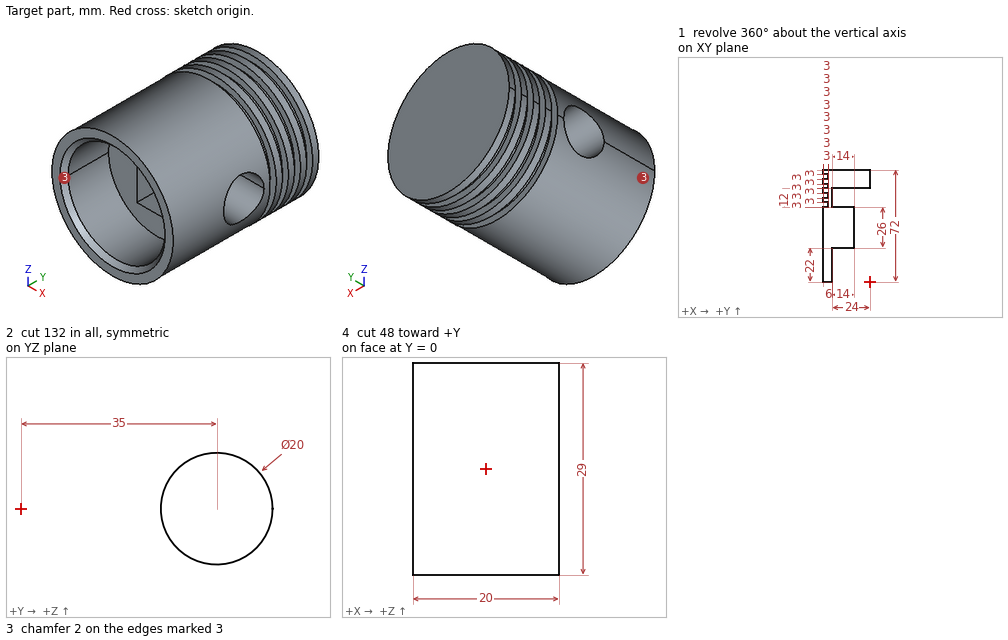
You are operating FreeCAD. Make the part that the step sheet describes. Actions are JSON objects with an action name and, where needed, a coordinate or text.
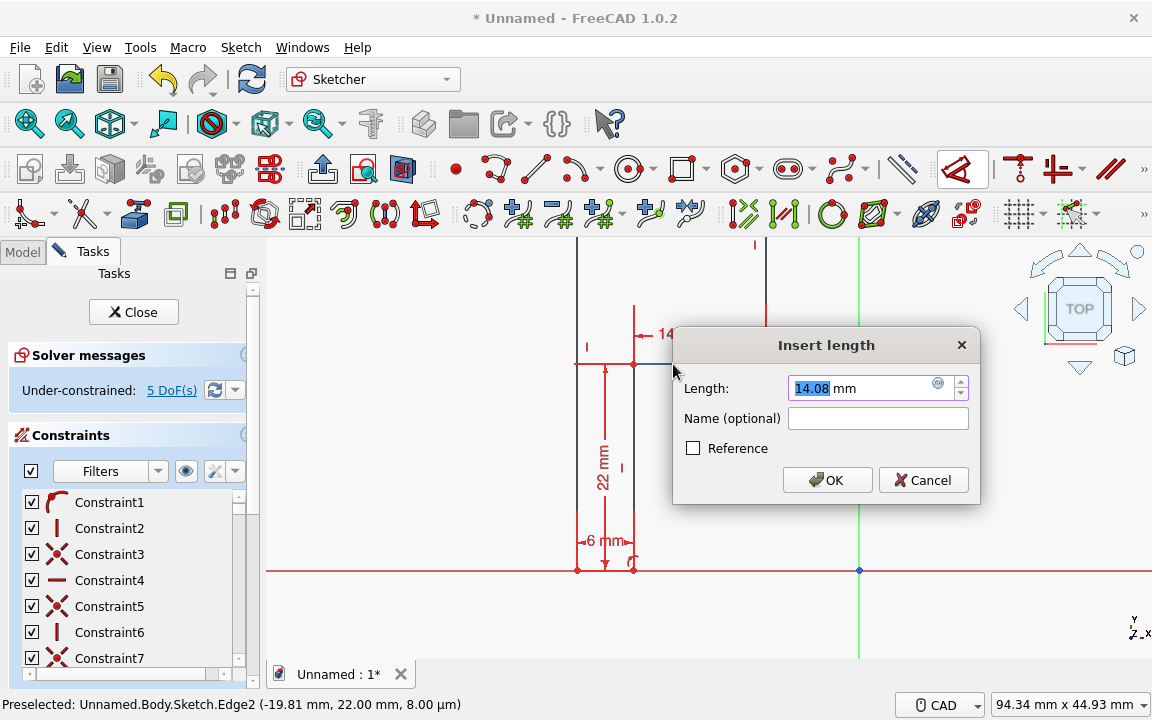
{"action": "type", "text": "14"}
{"action": "key", "text": "Return"}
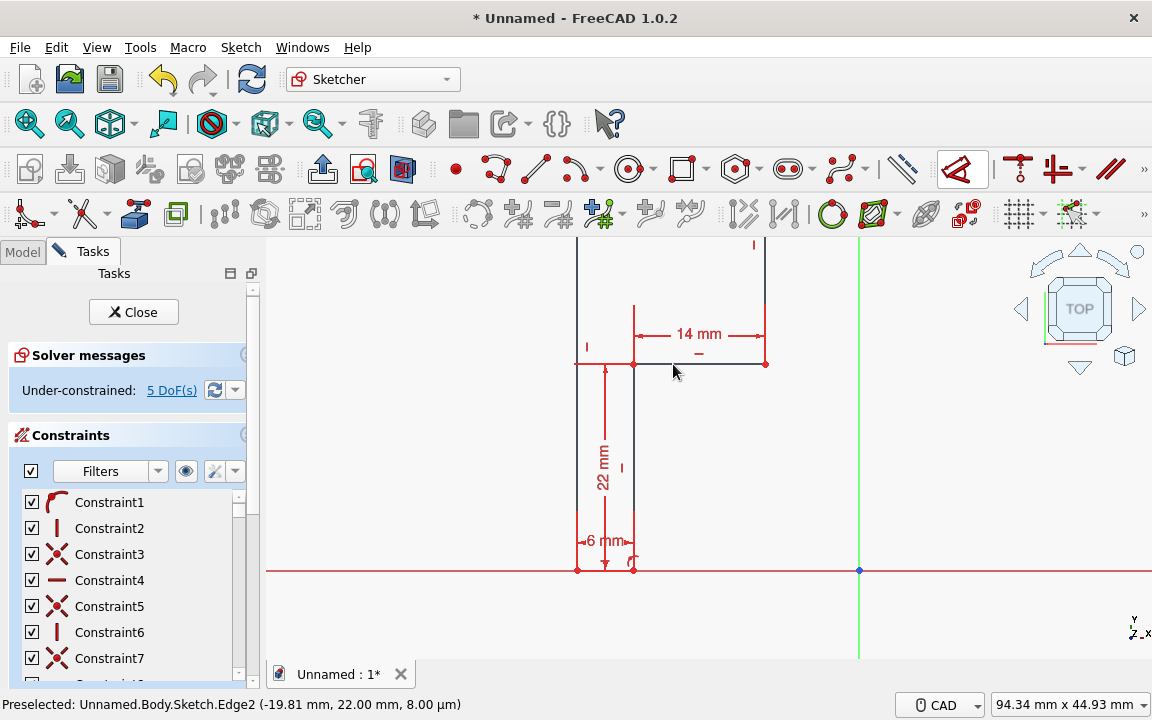
{"action": "left_click", "coordinate": [765, 292]}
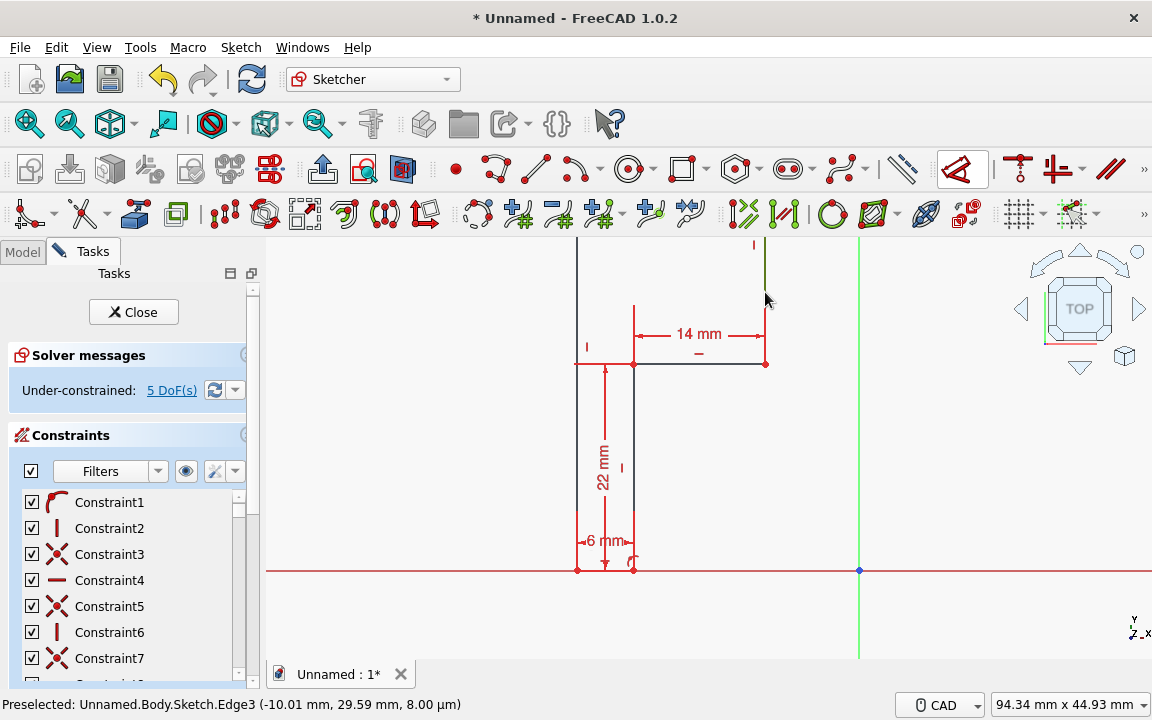
{"action": "left_click", "coordinate": [982, 170]}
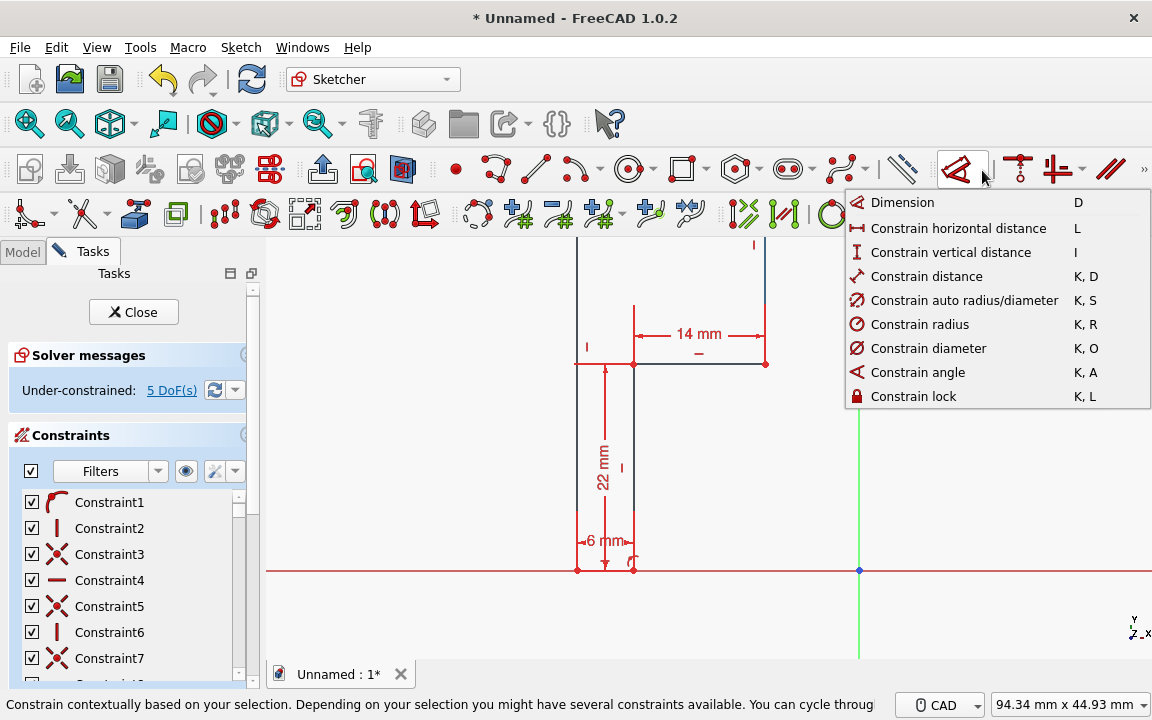
{"action": "left_click", "coordinate": [998, 252]}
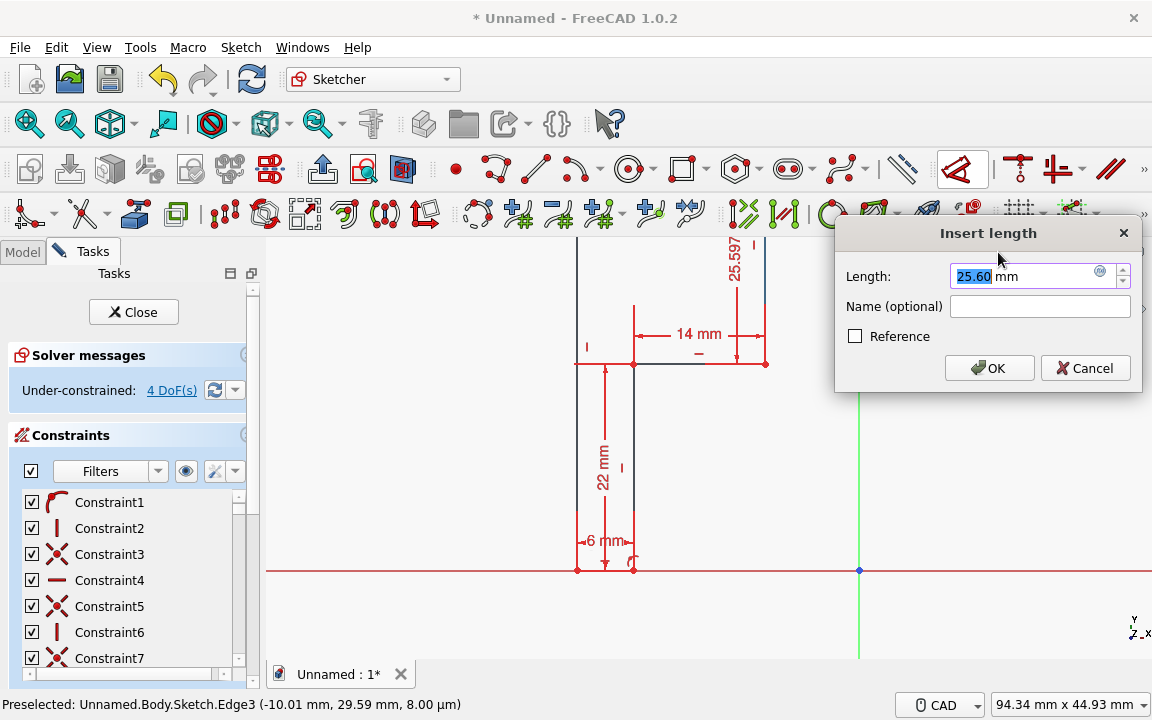
{"action": "type", "text": "26"}
{"action": "key", "text": "Return"}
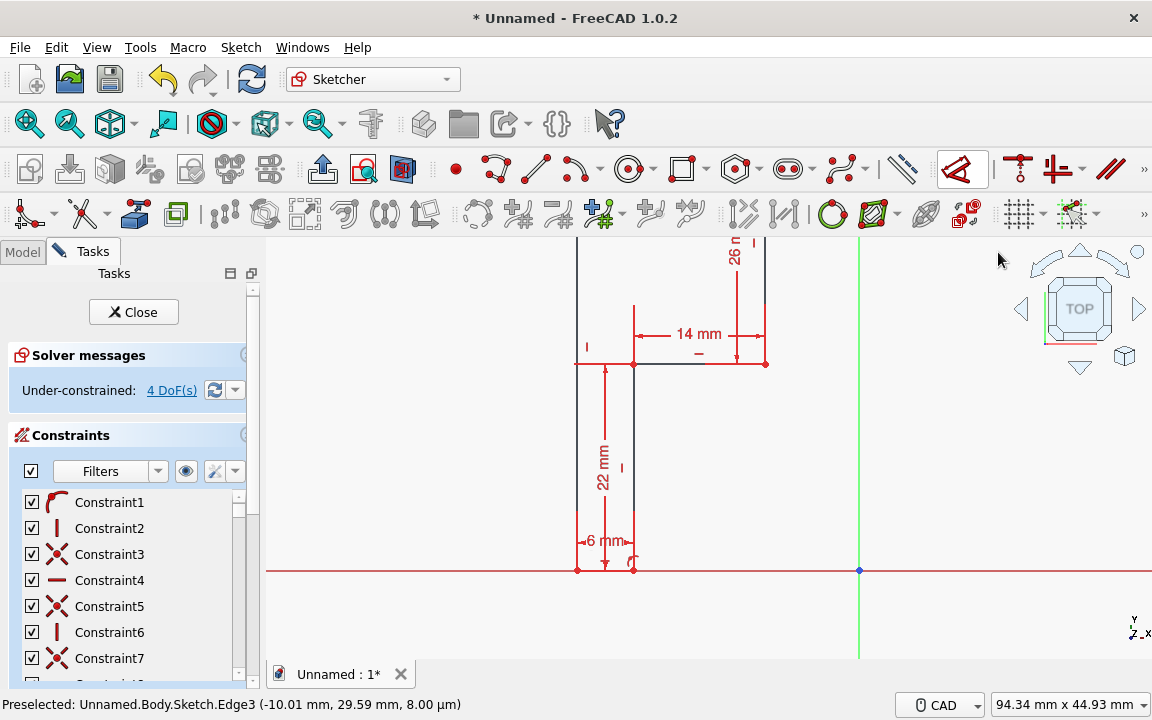
{"action": "scroll", "coordinate": [595, 573], "scroll_direction": "down", "scroll_amount": 5}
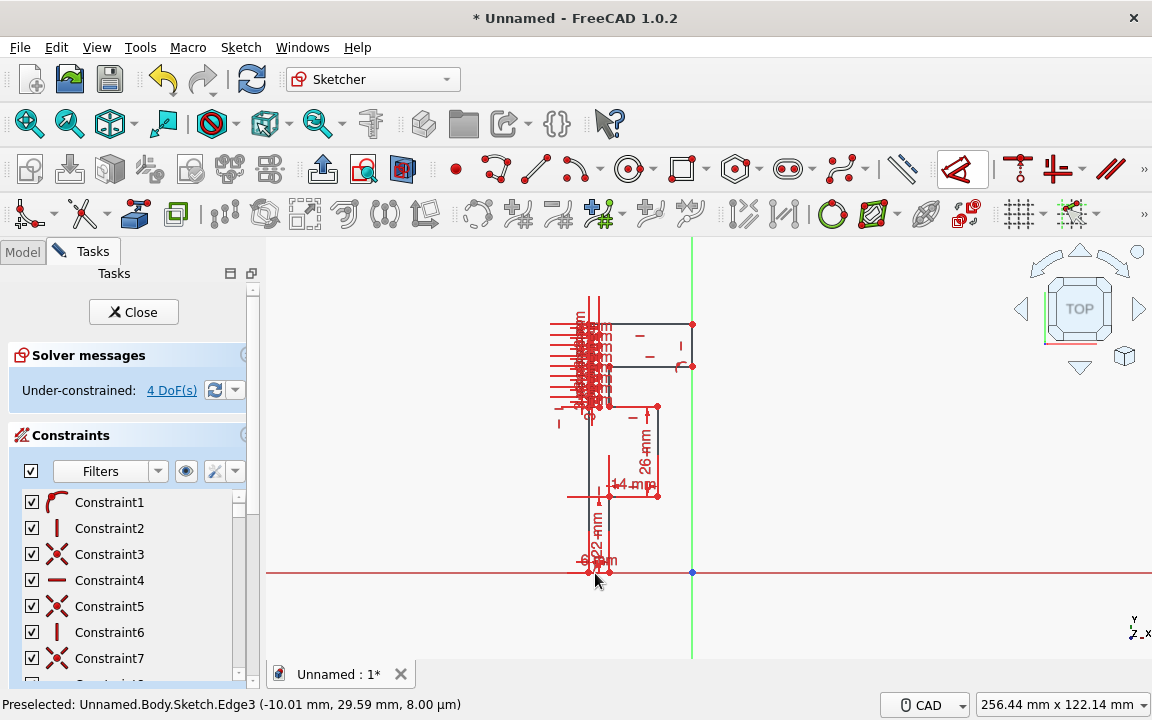
{"action": "left_click", "coordinate": [643, 407]}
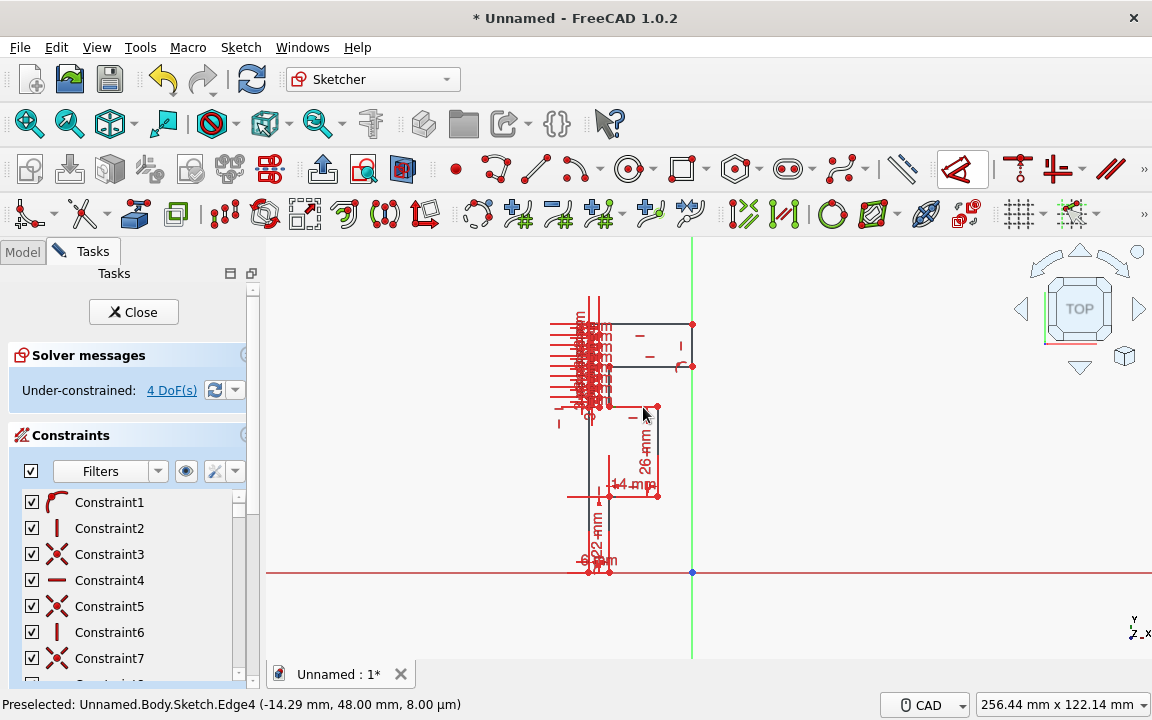
{"action": "left_click", "coordinate": [982, 170]}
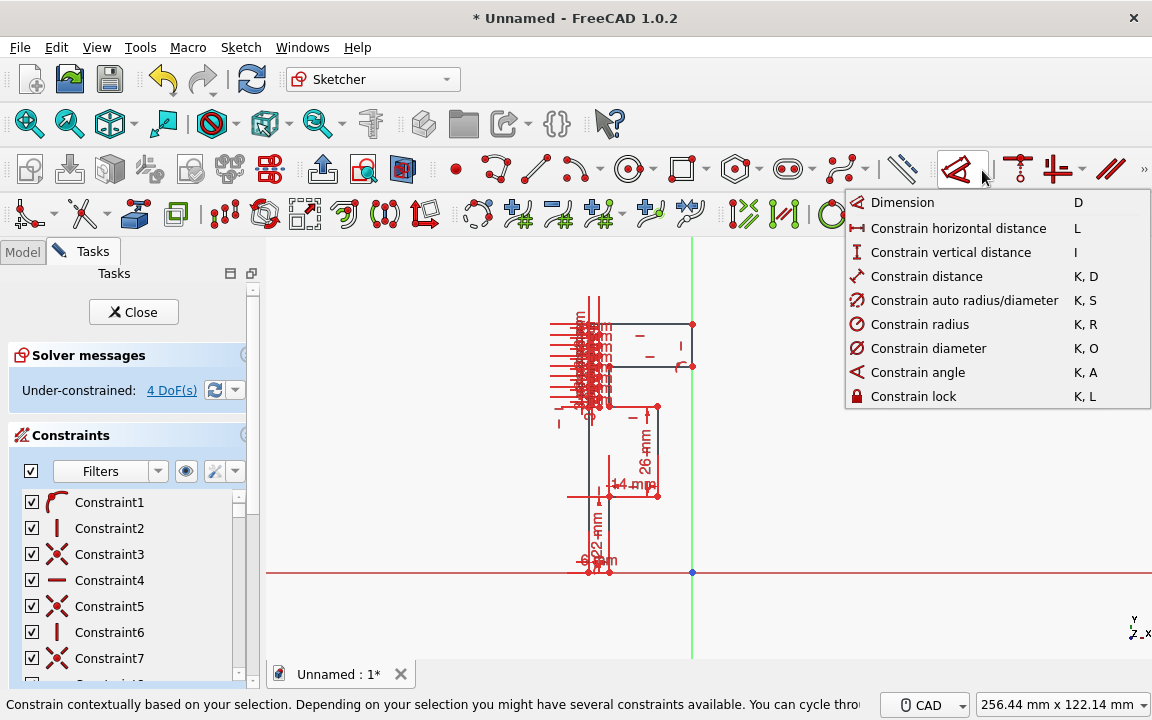
{"action": "left_click", "coordinate": [998, 228]}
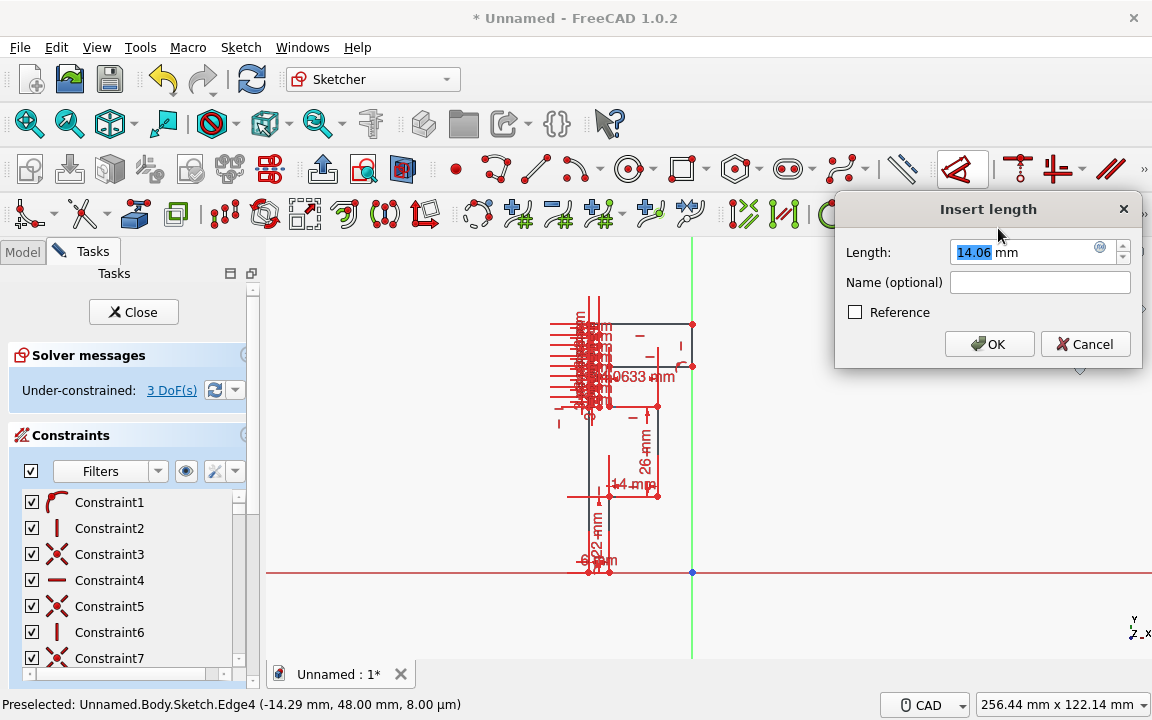
{"action": "type", "text": "14"}
{"action": "key", "text": "Return"}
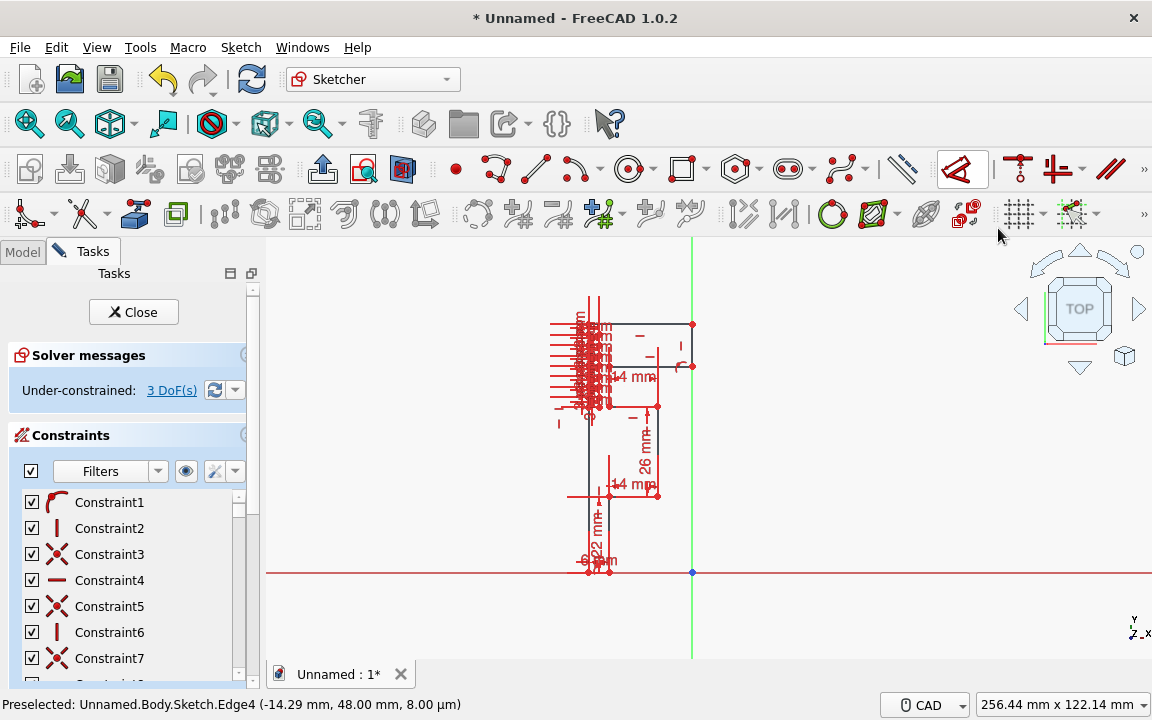
{"action": "scroll", "coordinate": [609, 395], "scroll_direction": "up", "scroll_amount": 2}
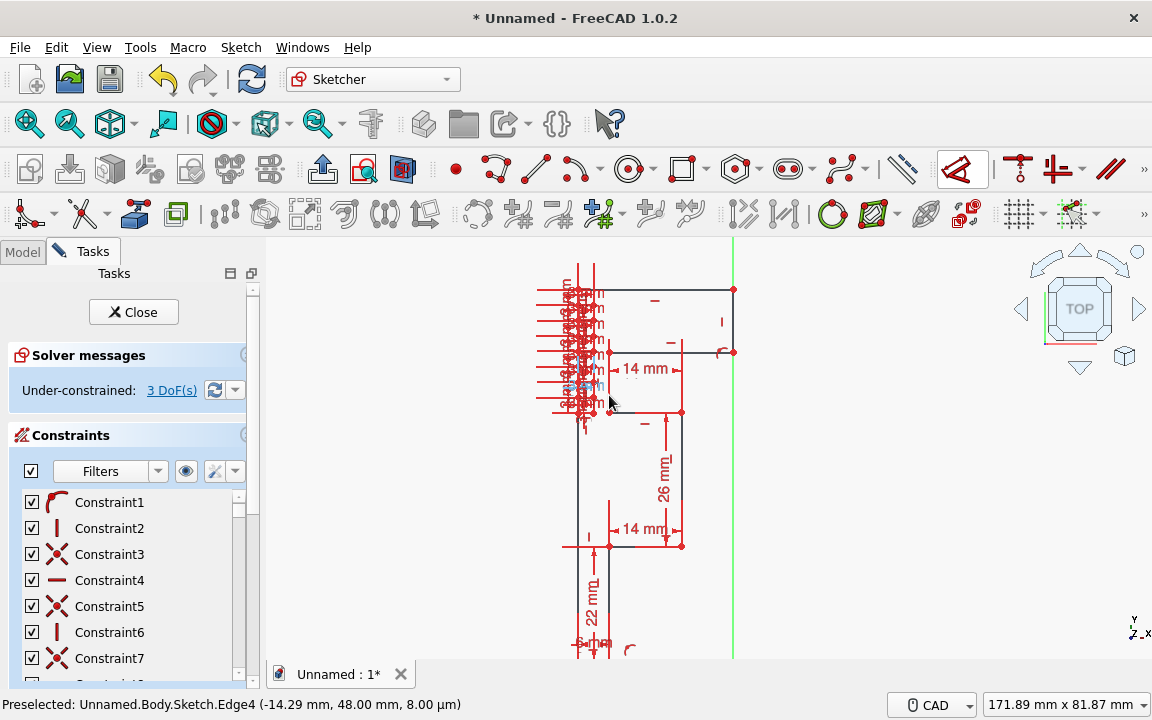
{"action": "left_click", "coordinate": [609, 395]}